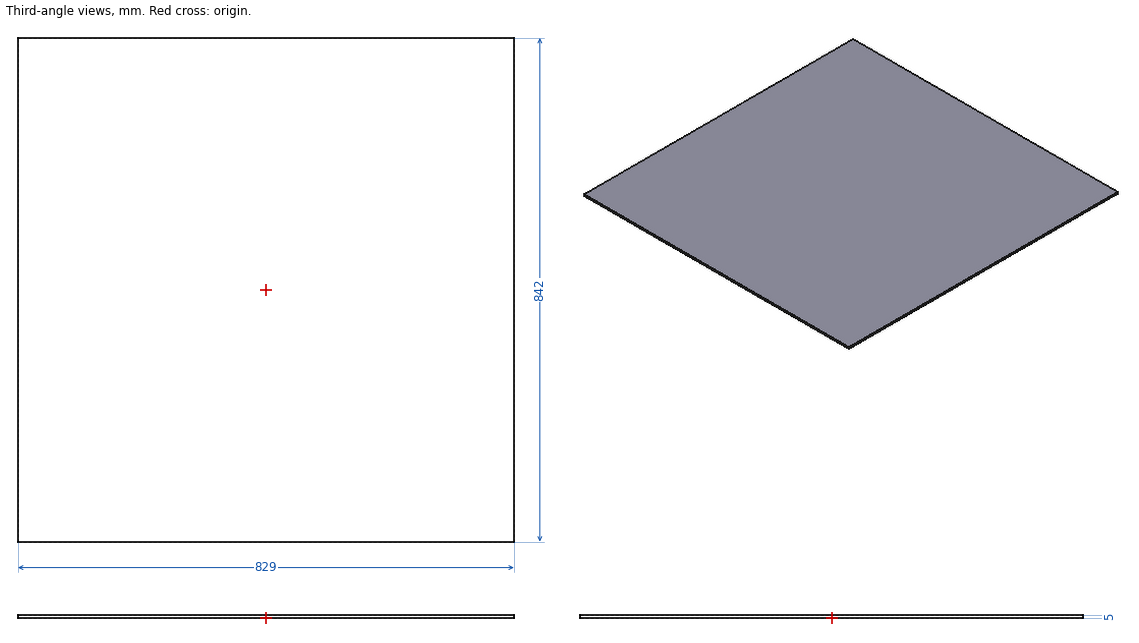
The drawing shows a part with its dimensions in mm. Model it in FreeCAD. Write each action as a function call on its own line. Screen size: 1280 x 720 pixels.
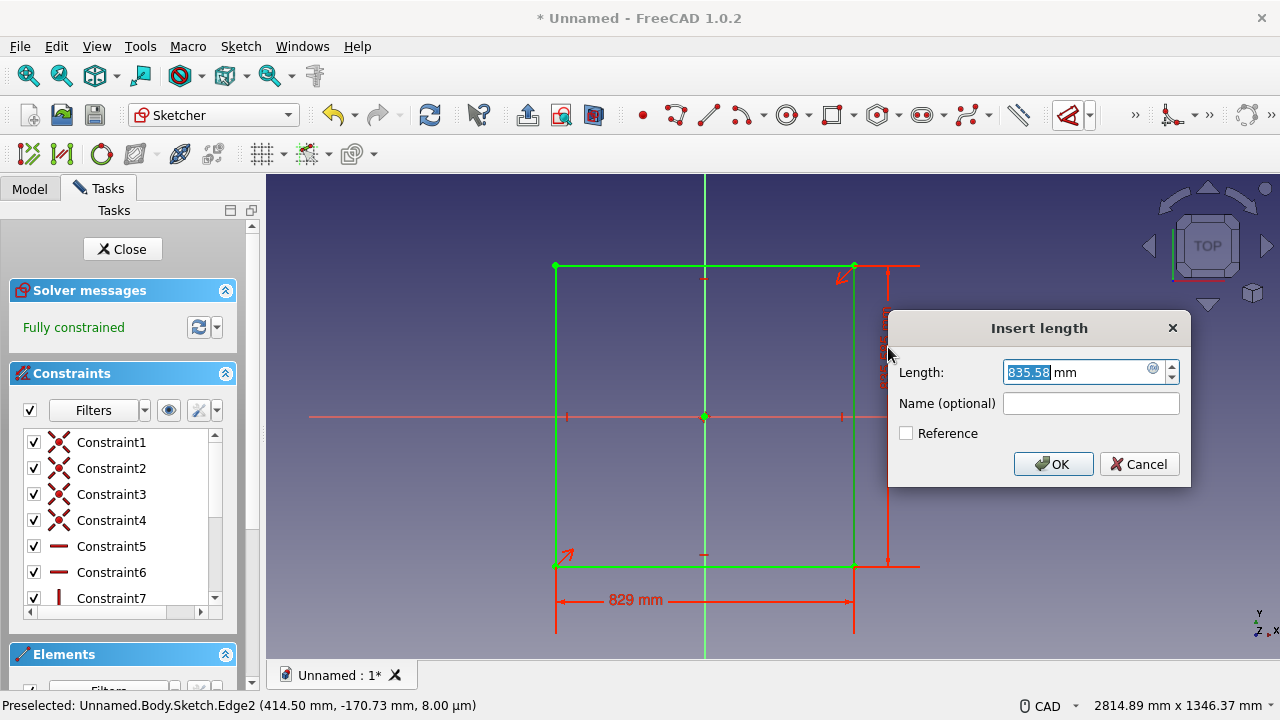
text(842)
key(Return)
key(Escape)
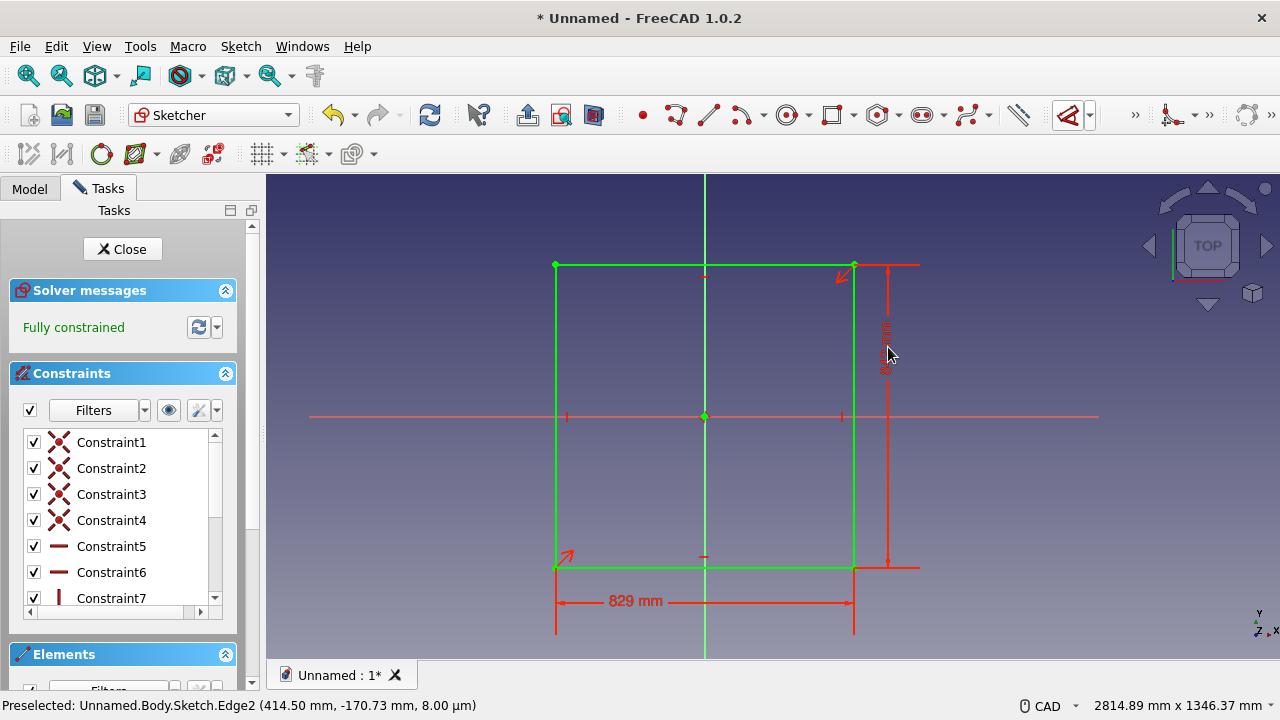
click(123, 249)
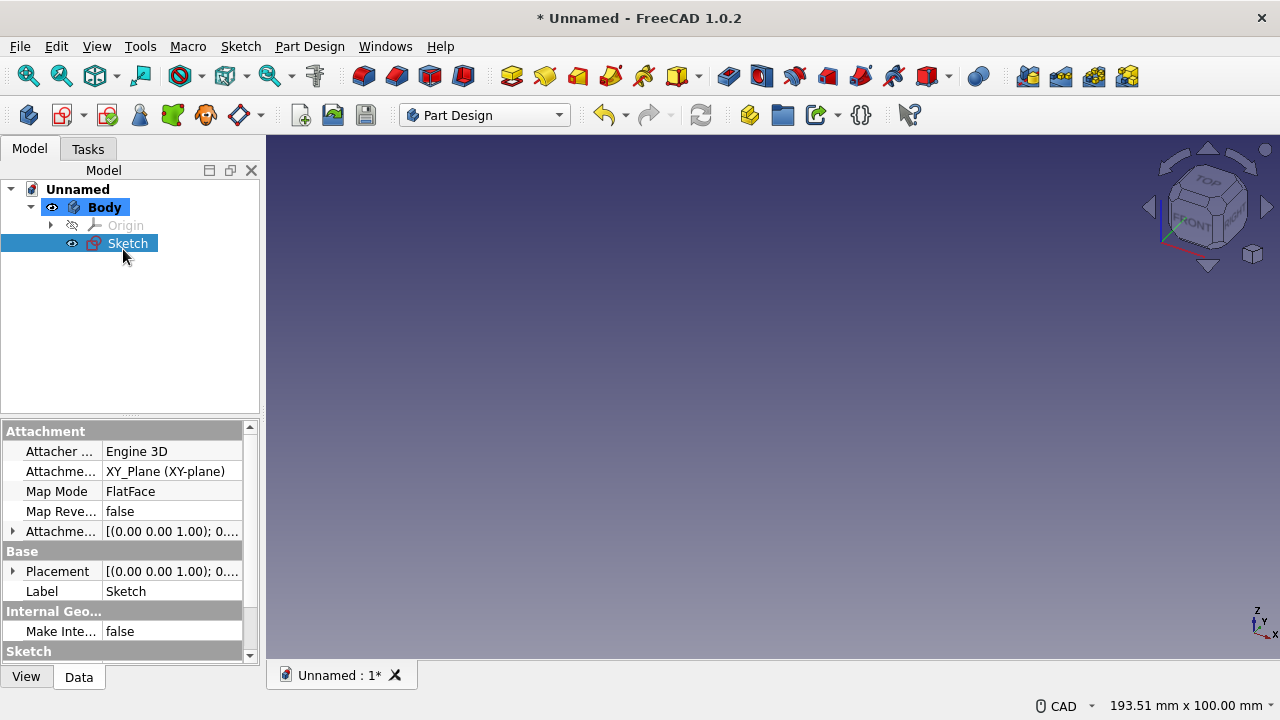
click(512, 76)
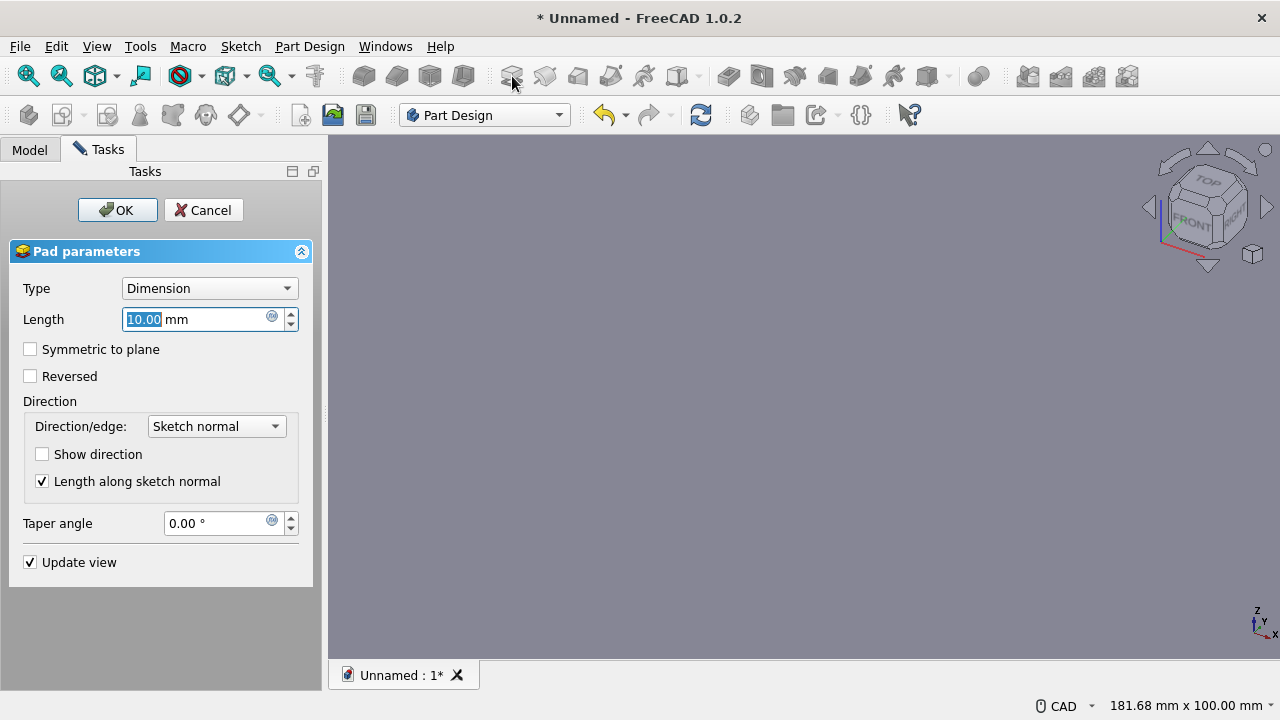
text(5)
key(Tab)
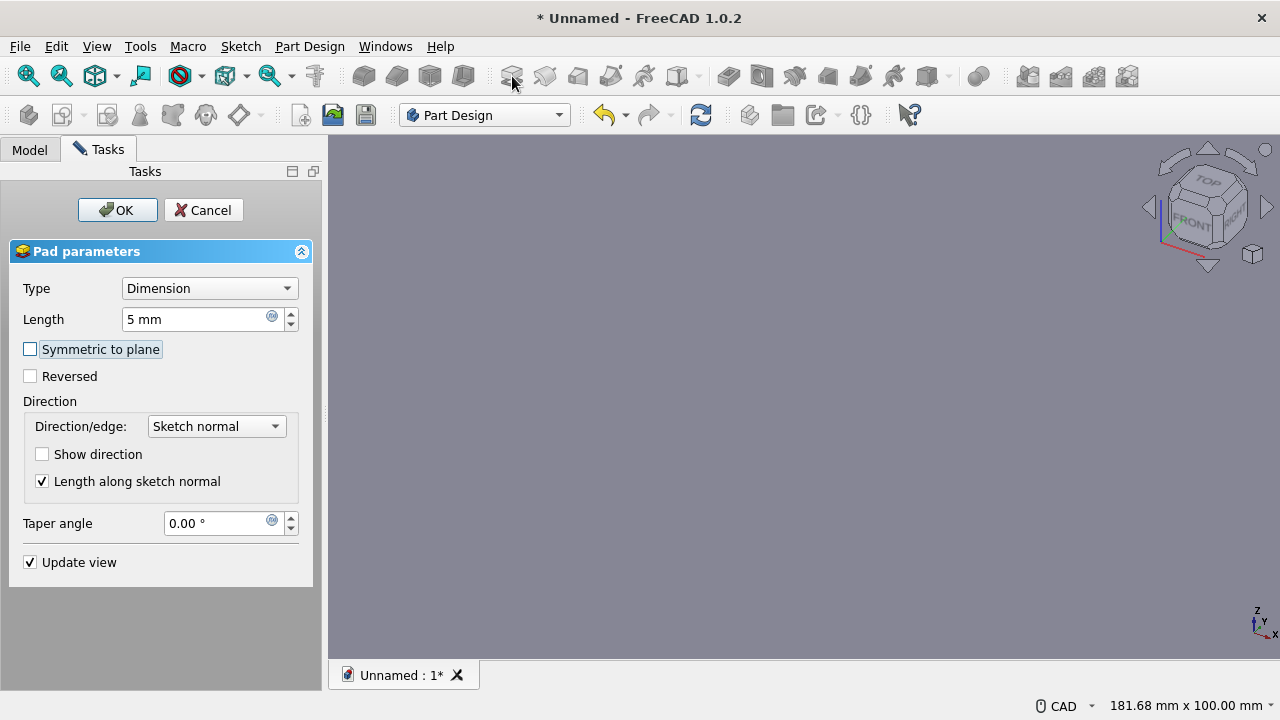
click(118, 210)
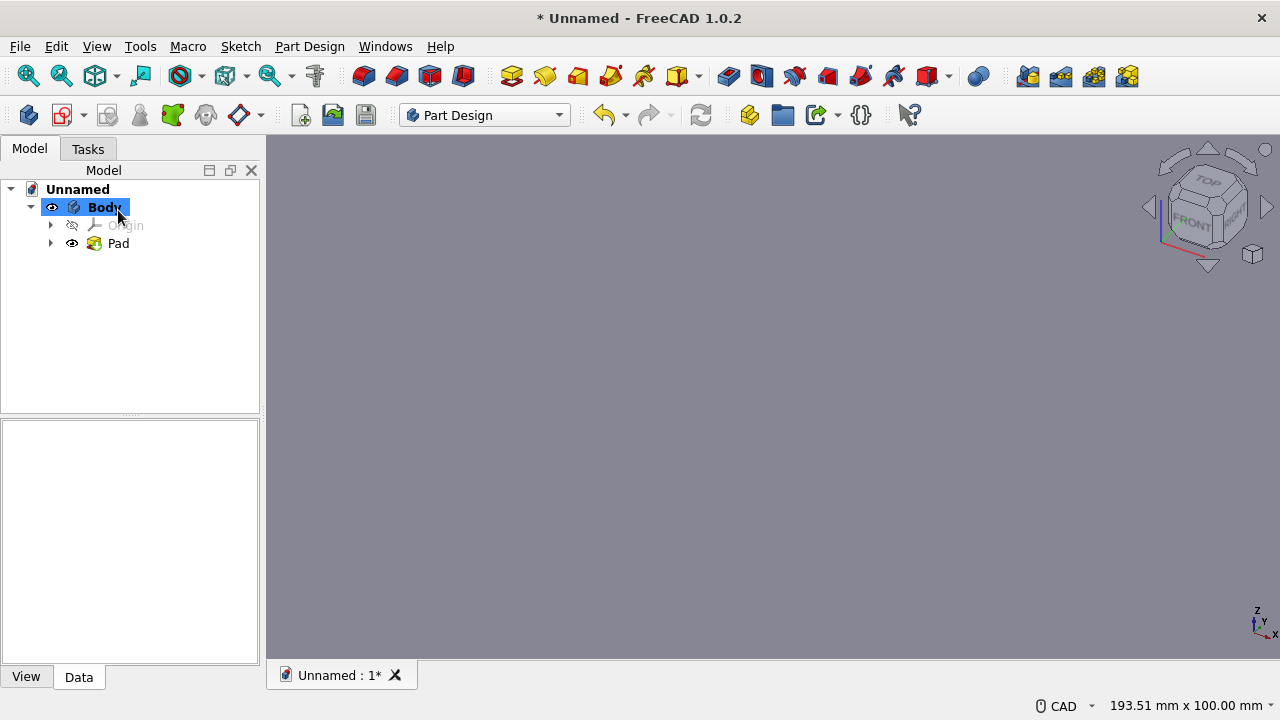
key(0)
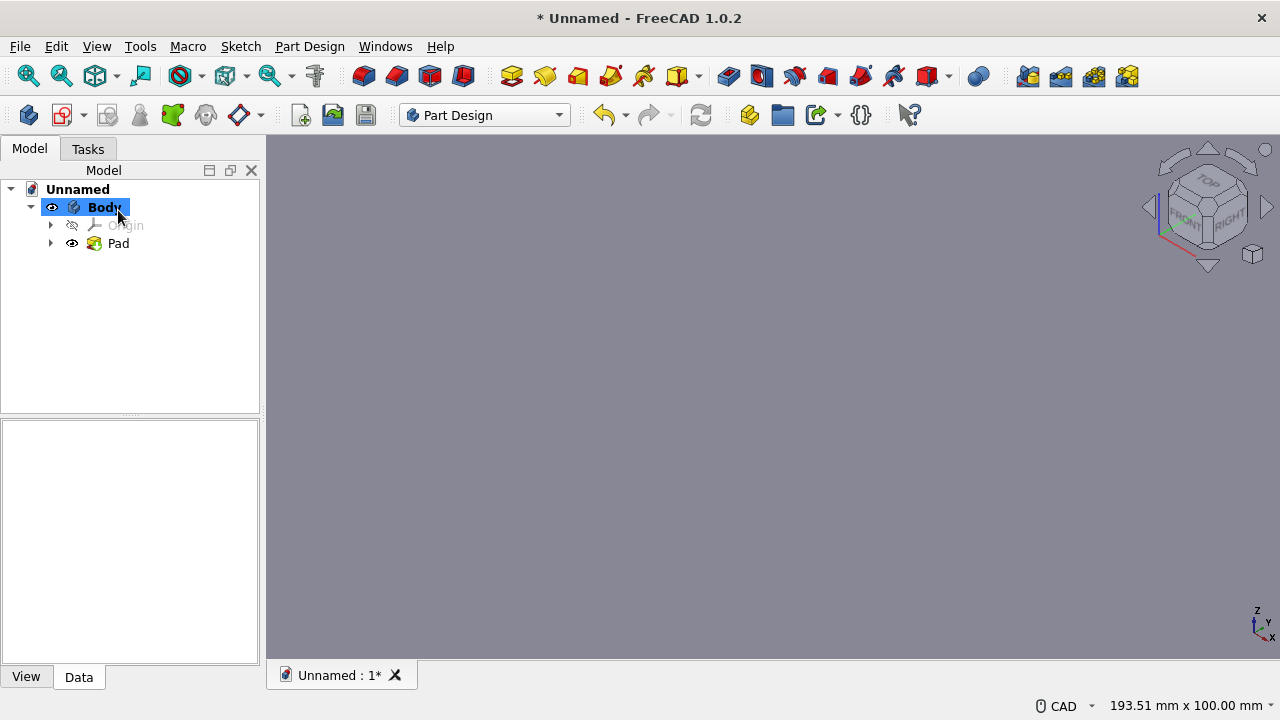
key(v)
key(f)